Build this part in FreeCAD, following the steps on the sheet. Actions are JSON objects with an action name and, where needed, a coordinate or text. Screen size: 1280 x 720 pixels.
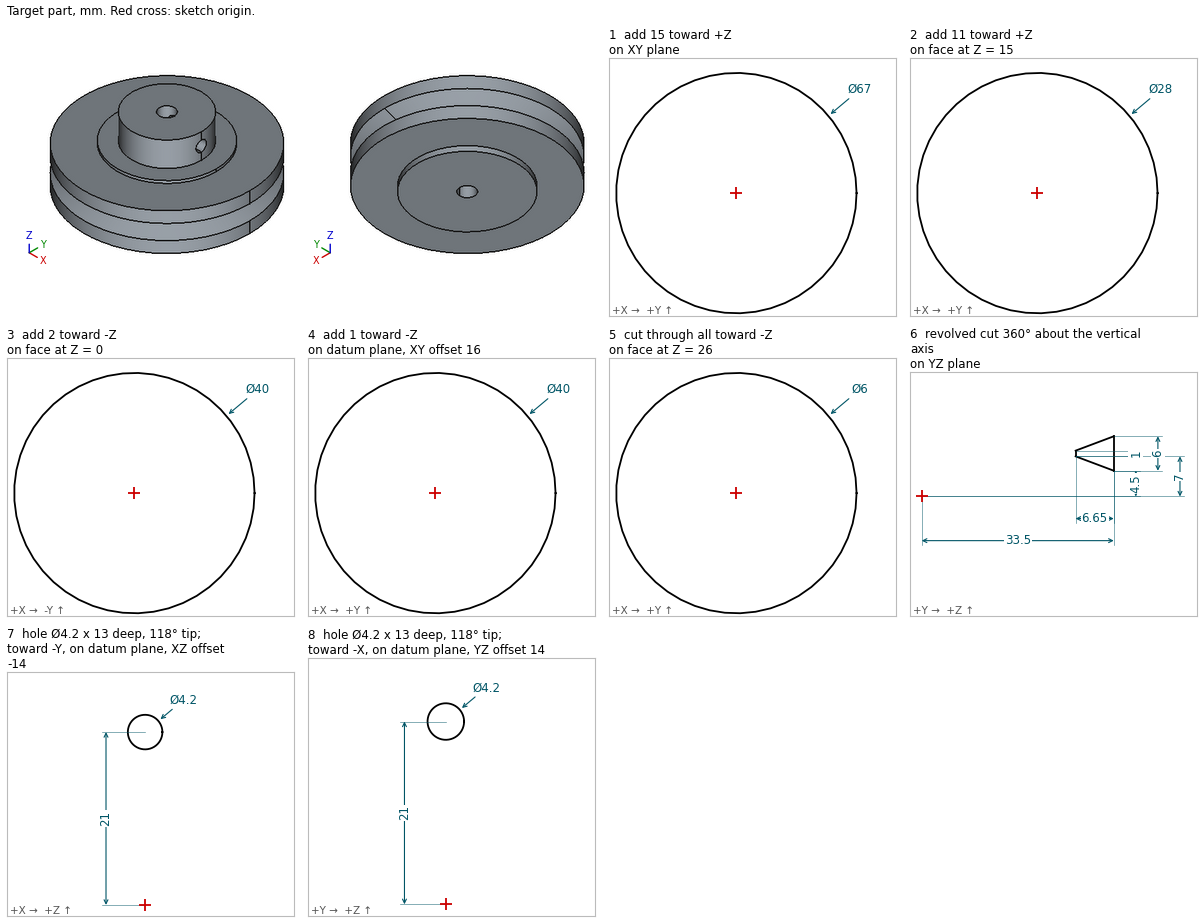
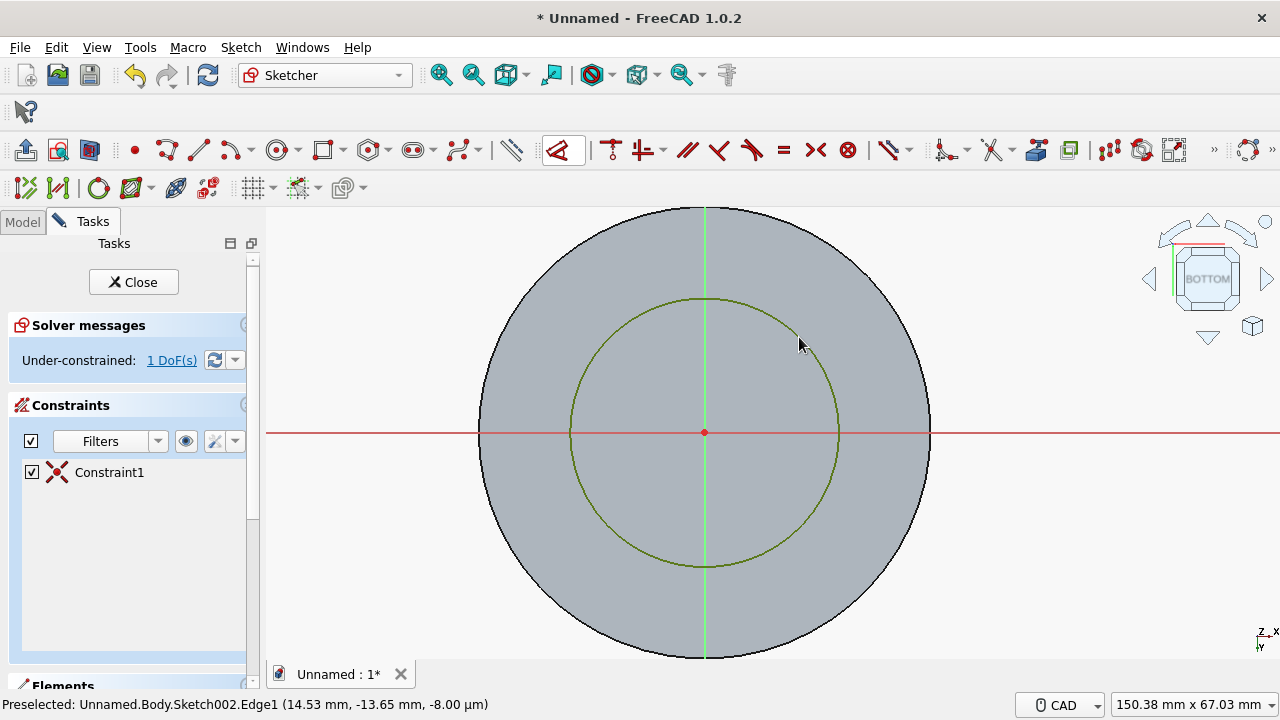
{"action": "left_click", "coordinate": [580, 150]}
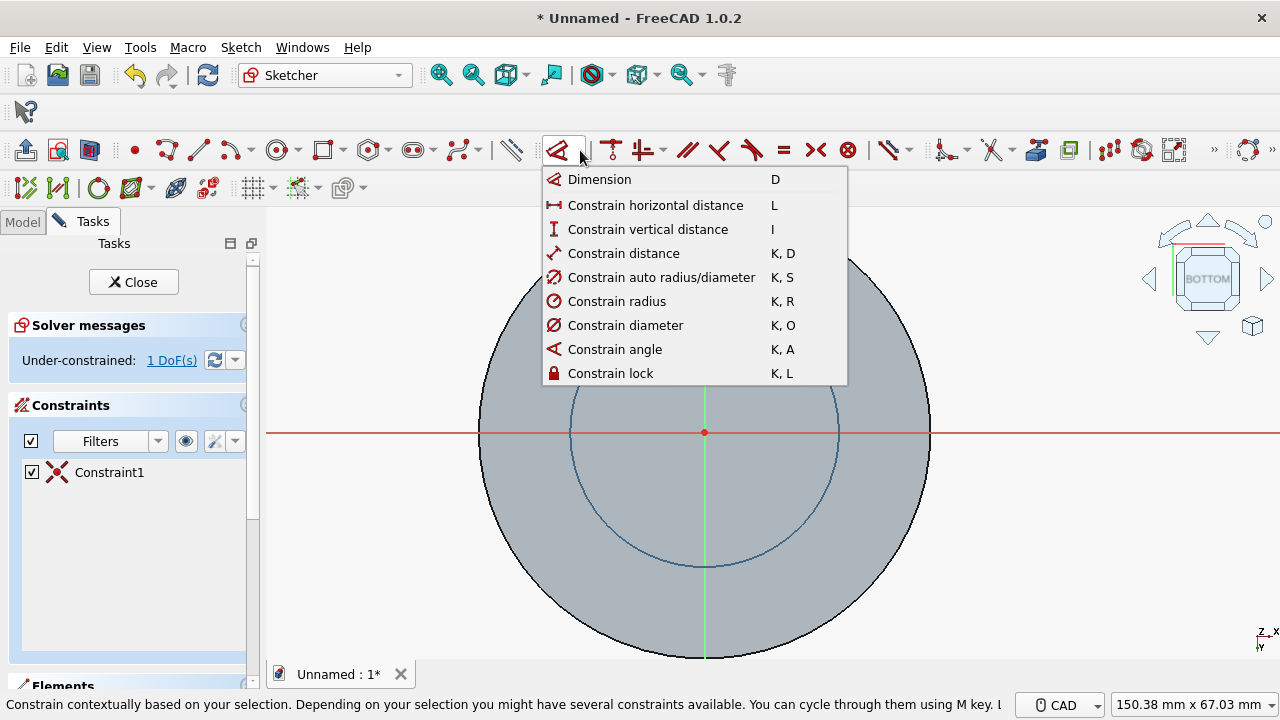
{"action": "left_click", "coordinate": [695, 325]}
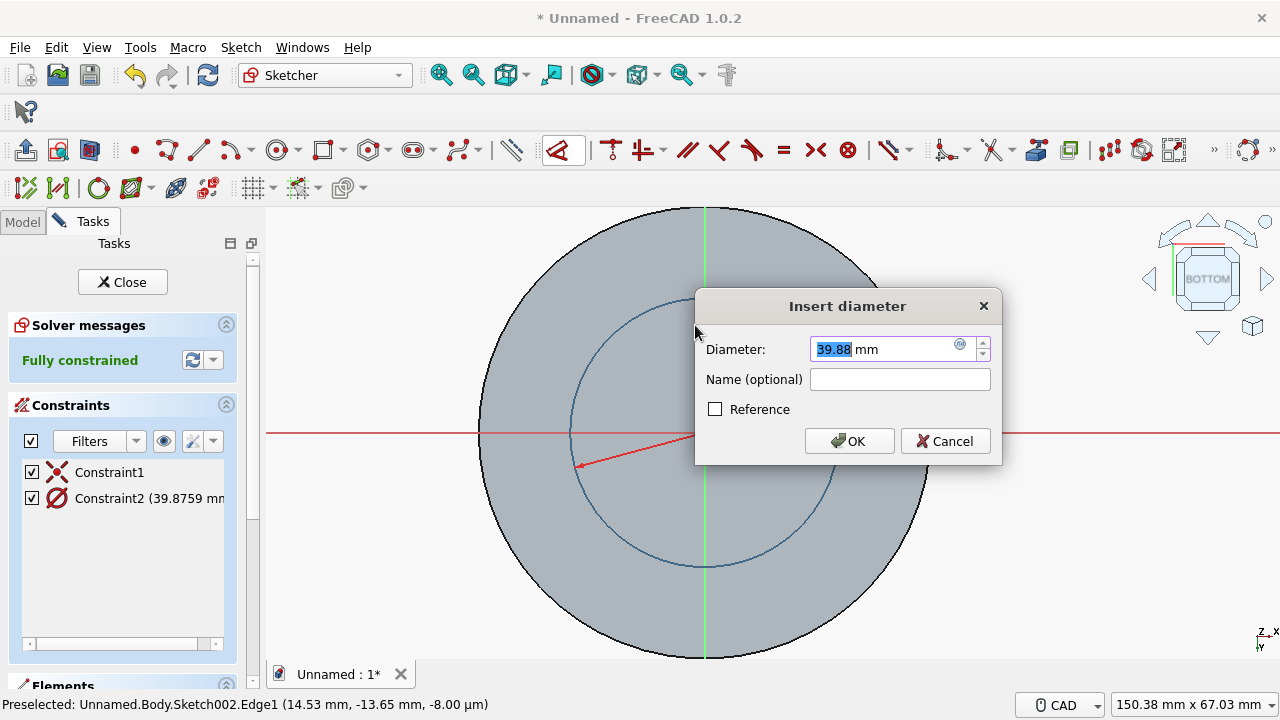
{"action": "type", "text": "40"}
{"action": "key", "text": "Return"}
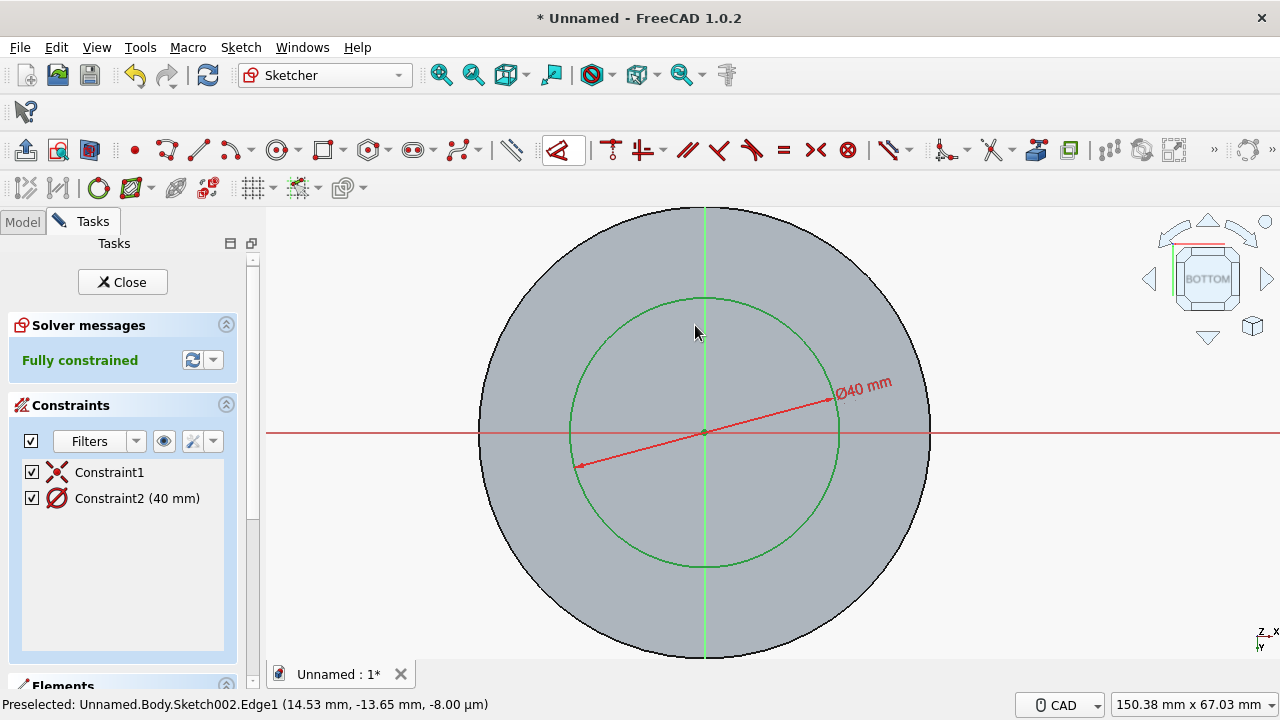
{"action": "left_click", "coordinate": [123, 282]}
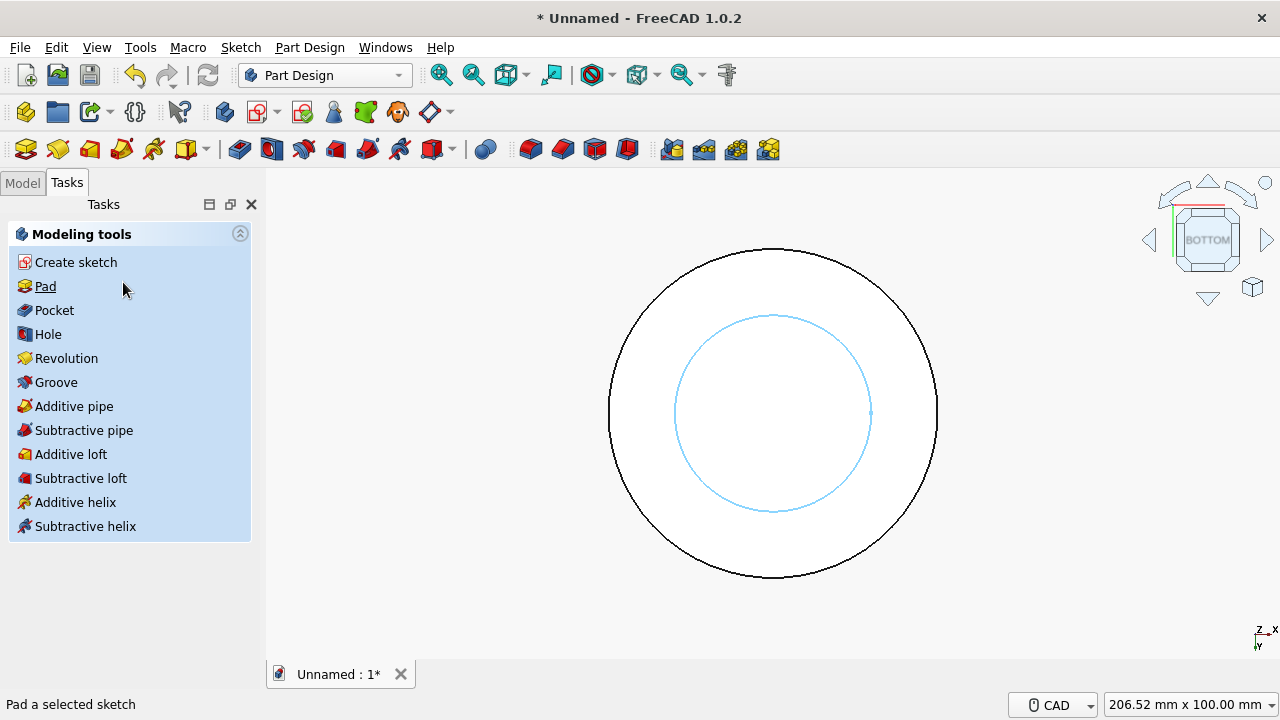
{"action": "left_click", "coordinate": [26, 150]}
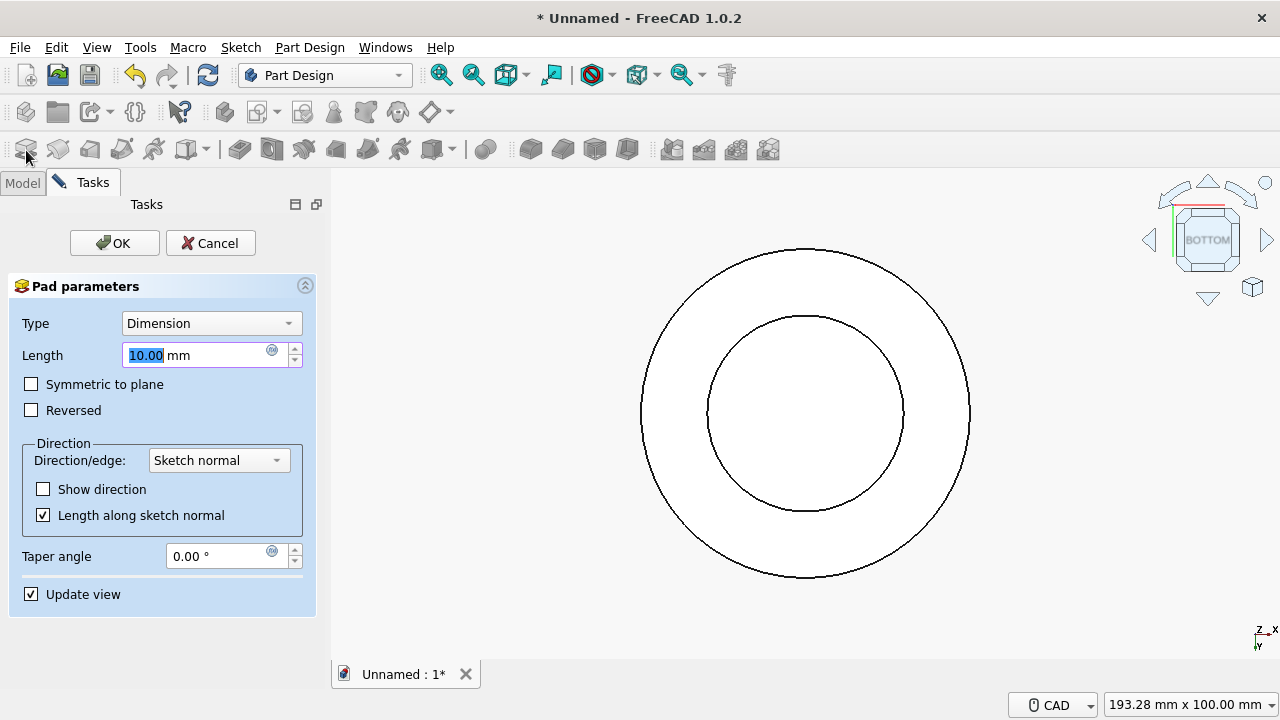
{"action": "type", "text": "2"}
{"action": "key", "text": "Tab"}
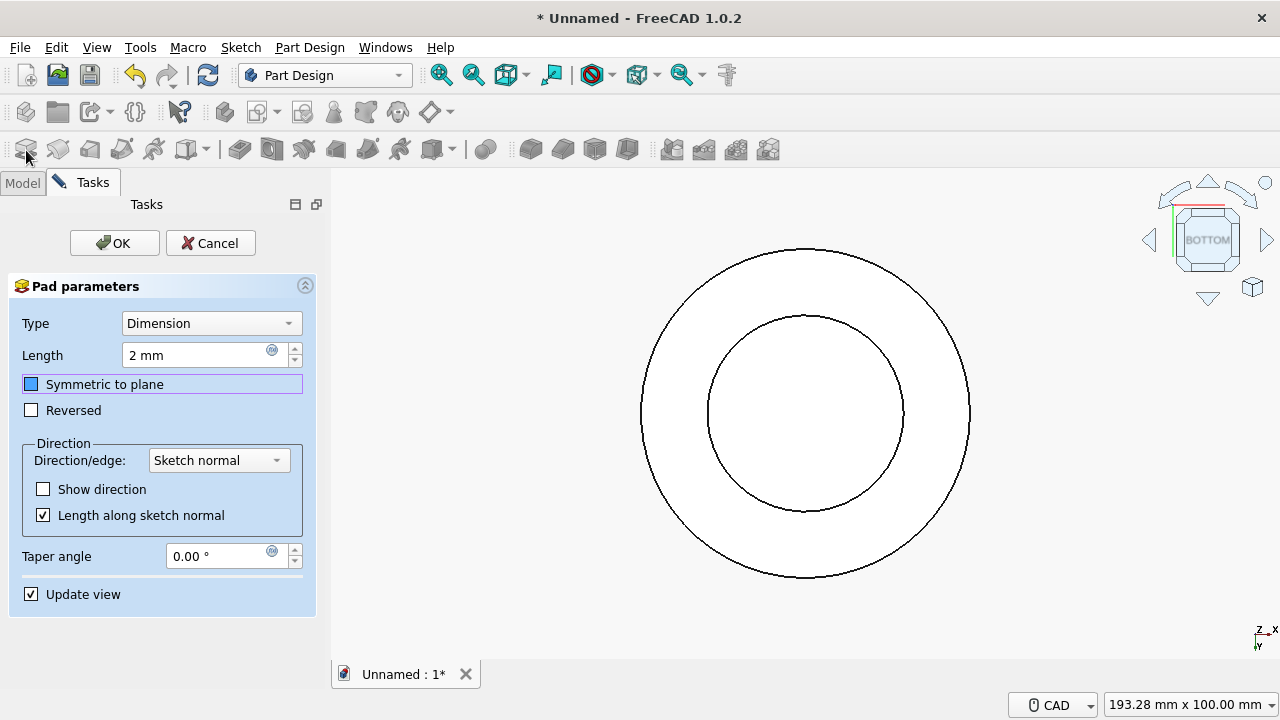
{"action": "left_click", "coordinate": [115, 243]}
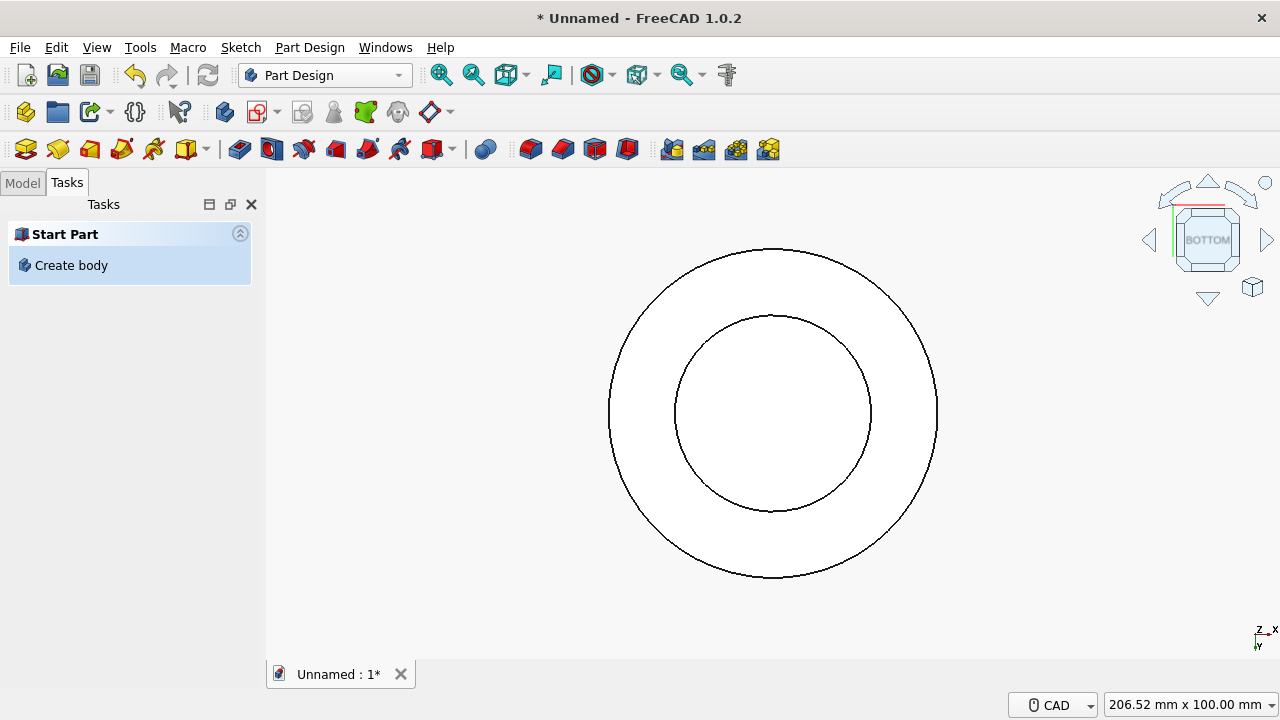
{"action": "left_click", "coordinate": [23, 182]}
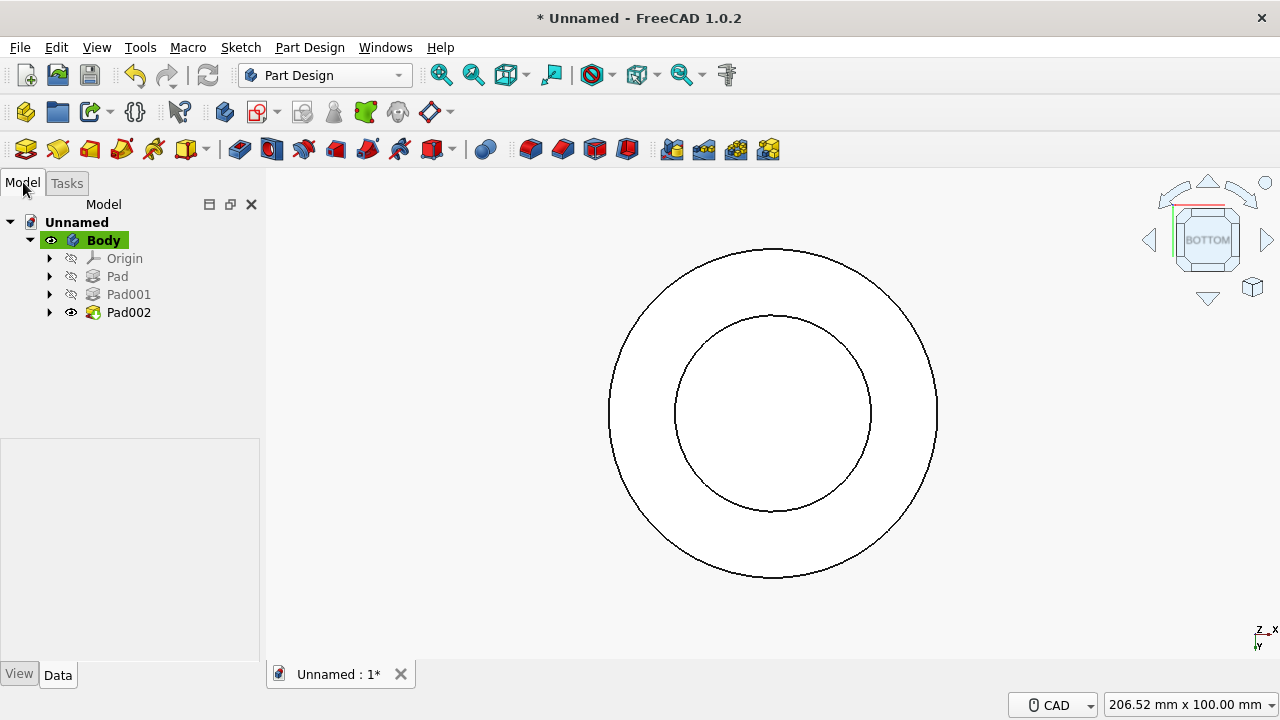
{"action": "left_click", "coordinate": [50, 258]}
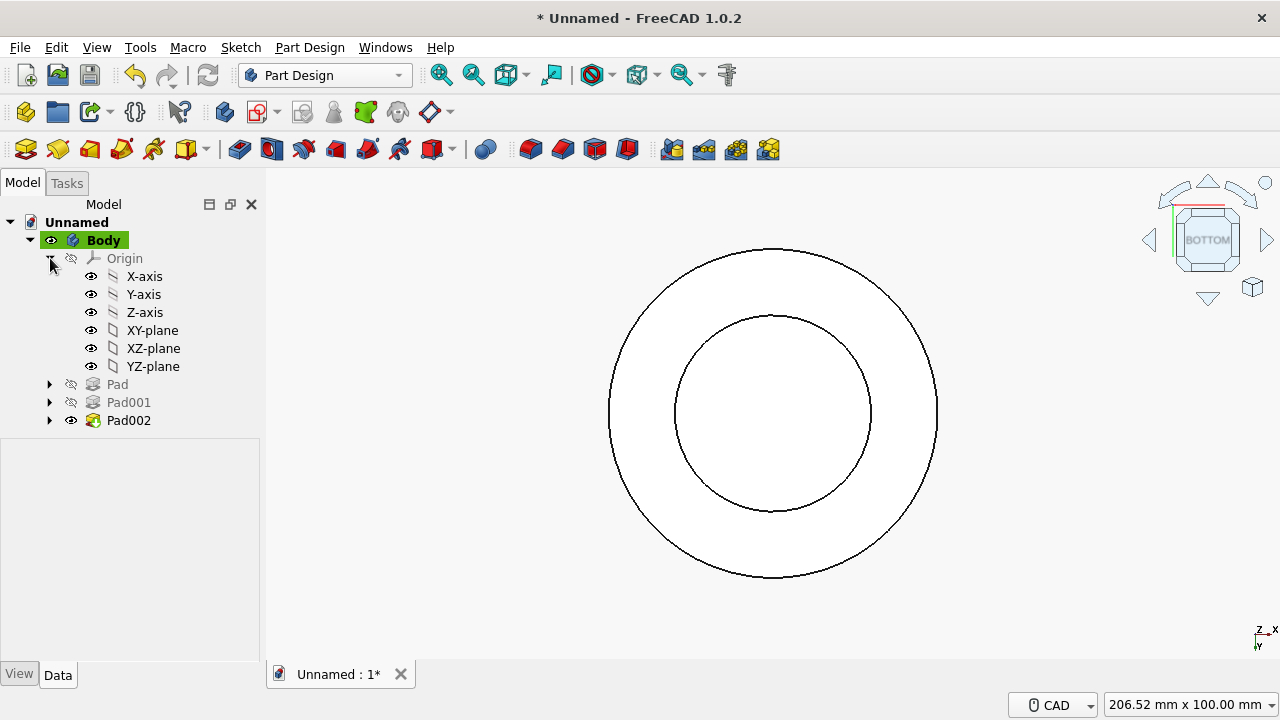
{"action": "left_click", "coordinate": [136, 330]}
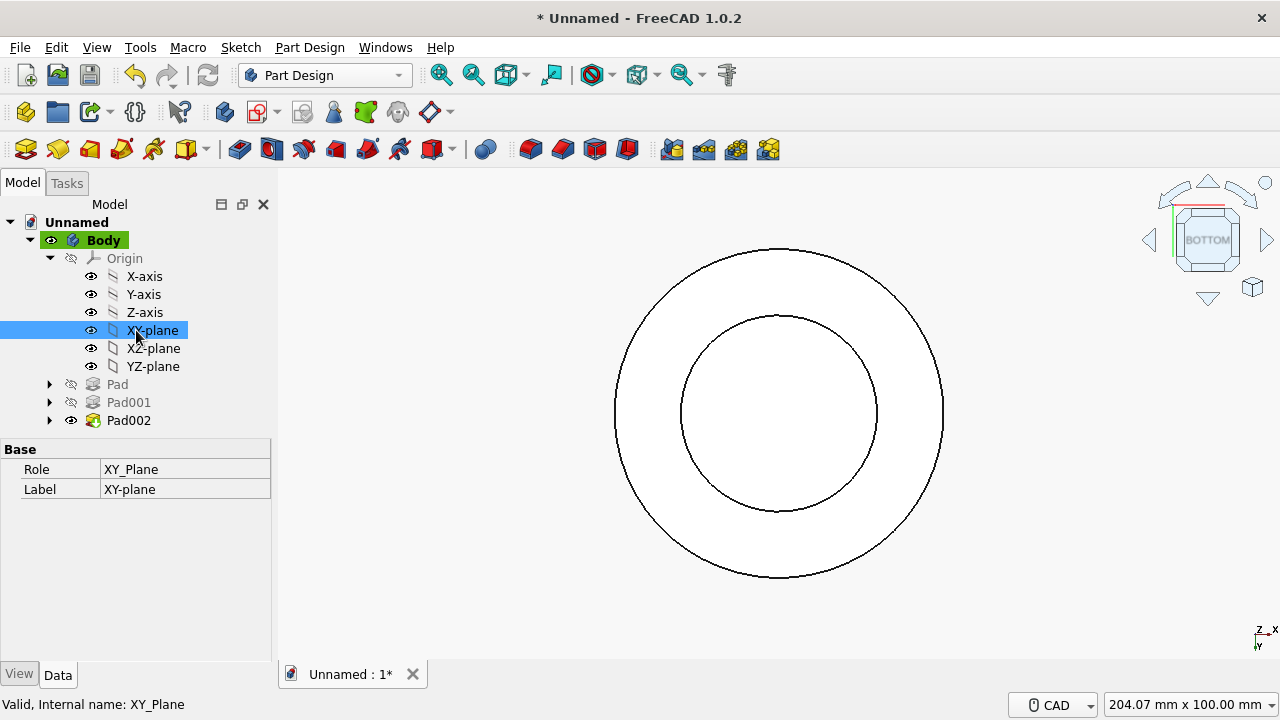
{"action": "left_click", "coordinate": [430, 112]}